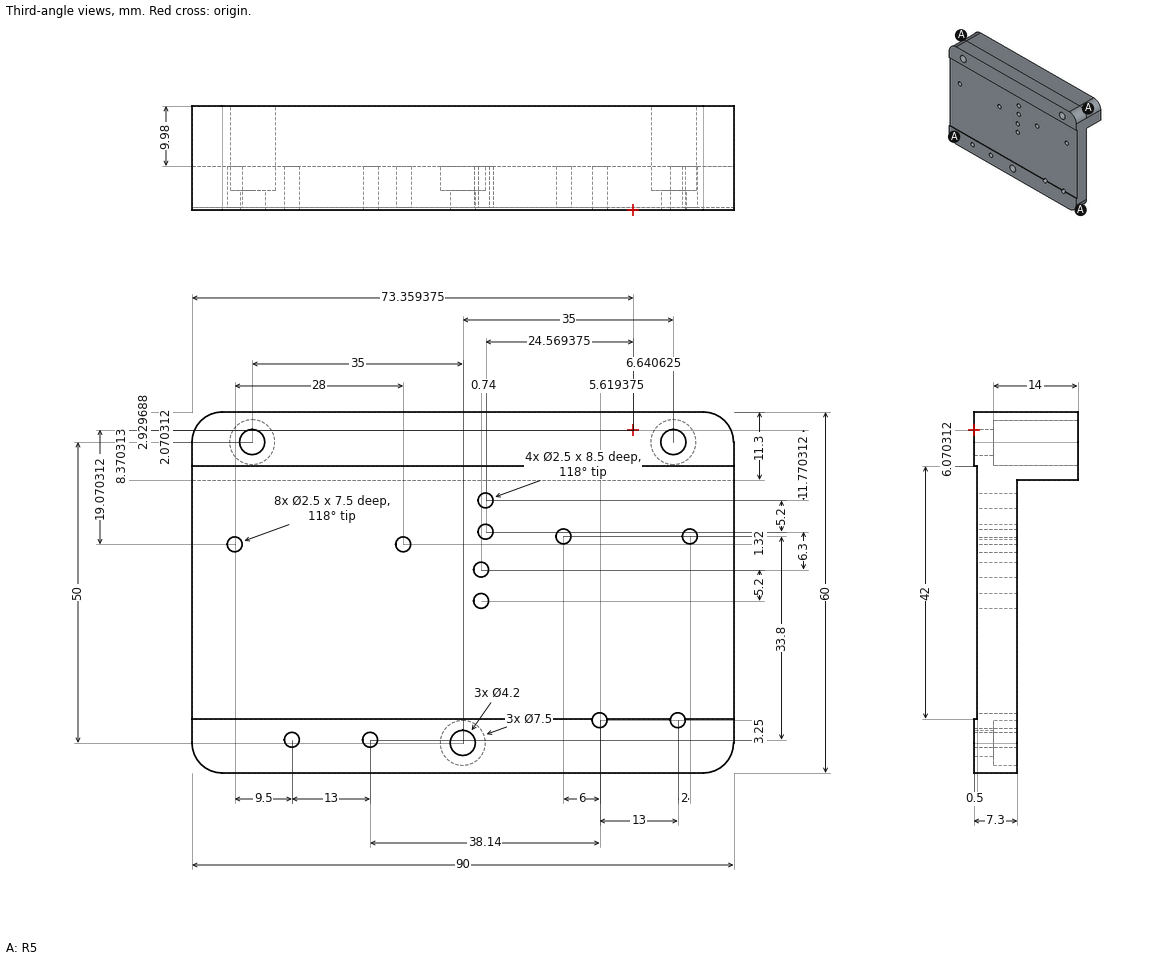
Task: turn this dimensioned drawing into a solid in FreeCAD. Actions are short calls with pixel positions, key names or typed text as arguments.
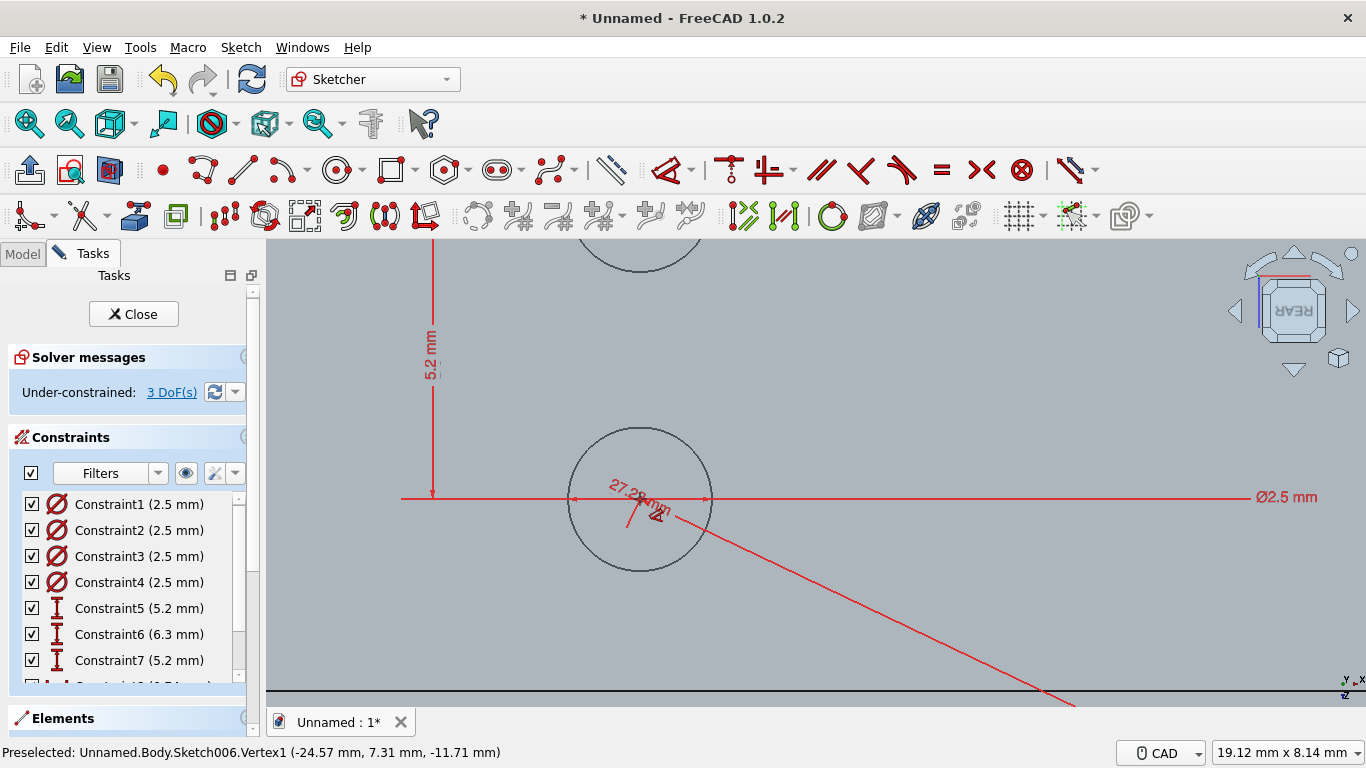
scroll(640, 504, down, 9)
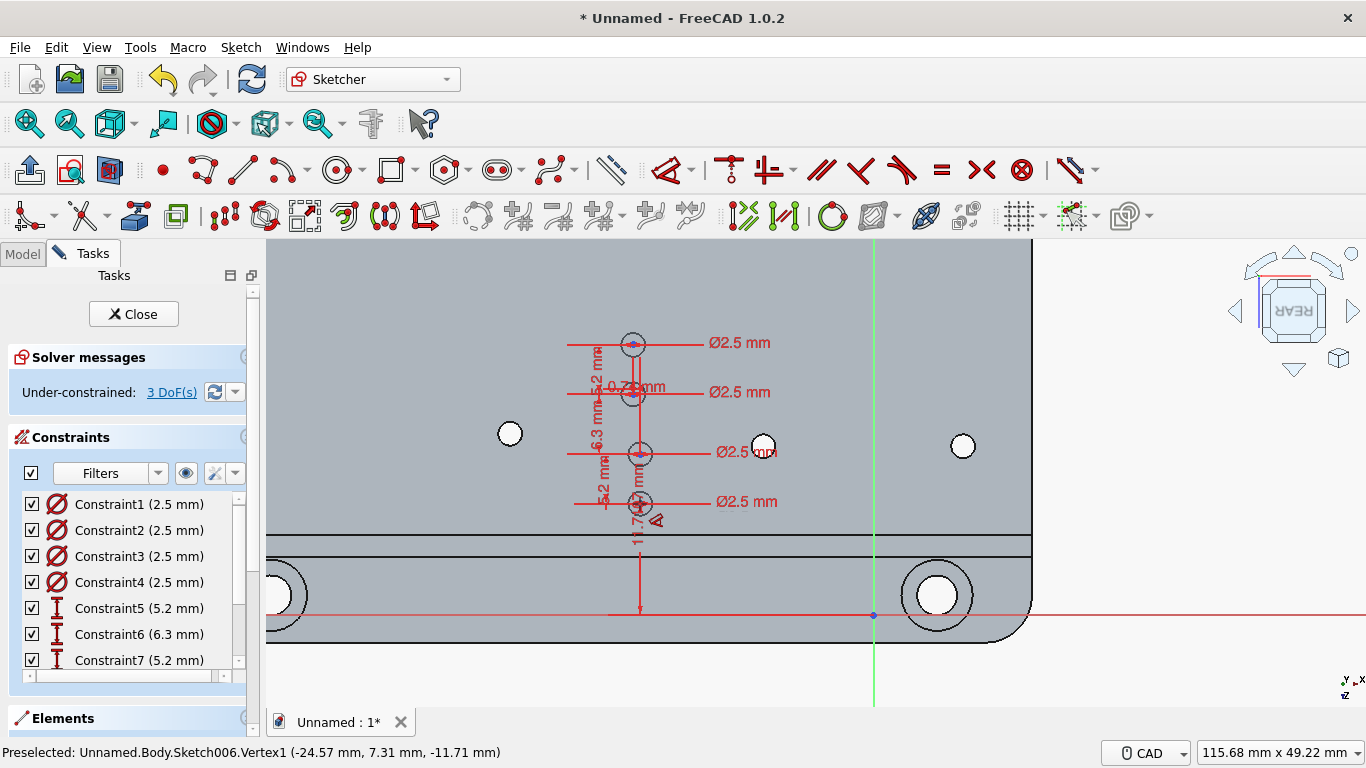
scroll(633, 394, up, 9)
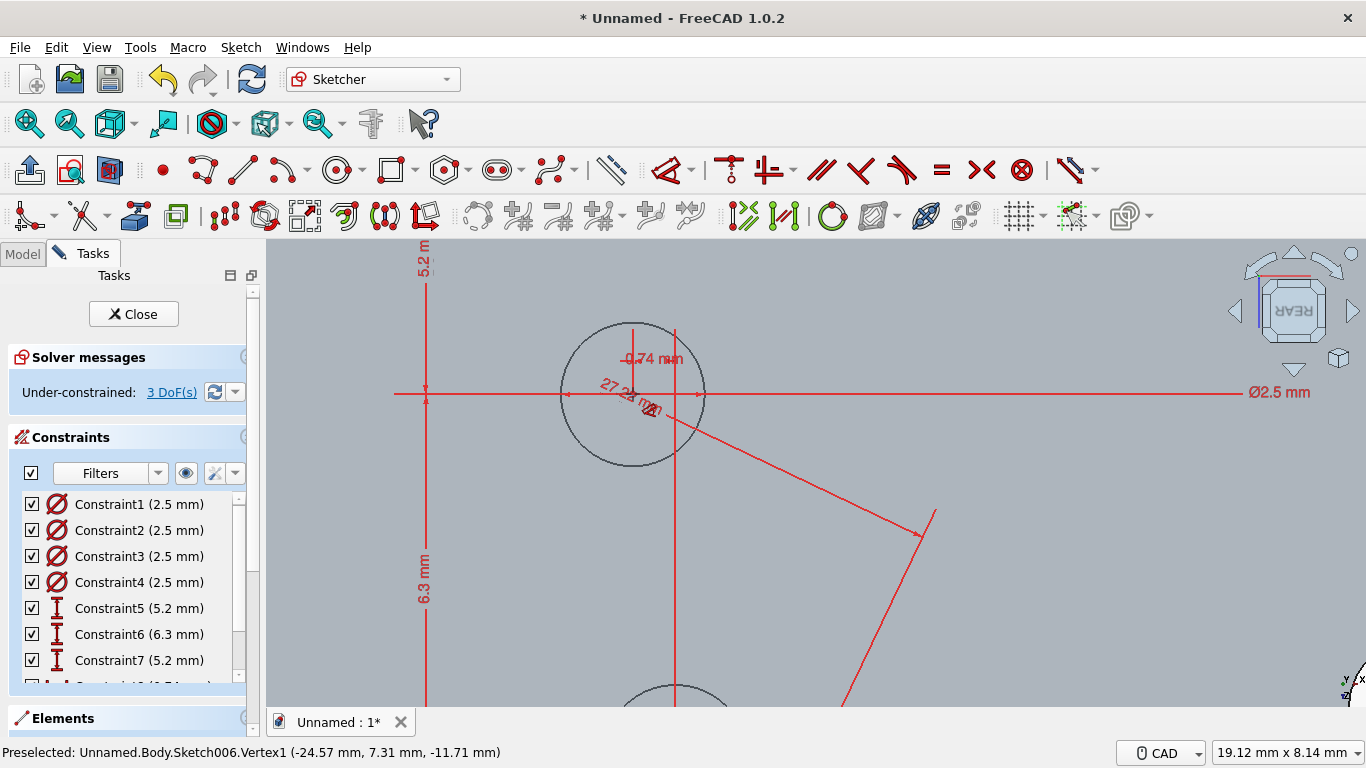
click(633, 394)
click(639, 336)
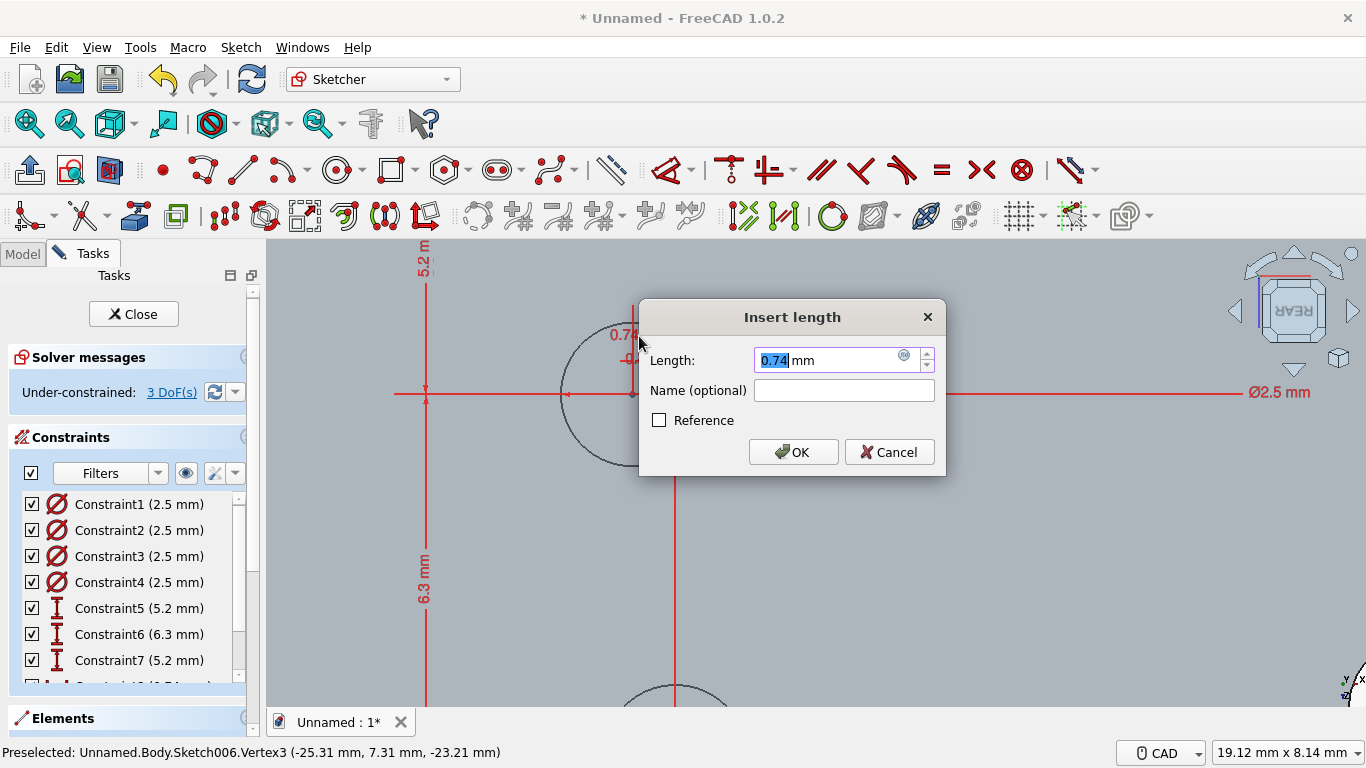
text(0.74)
key(Return)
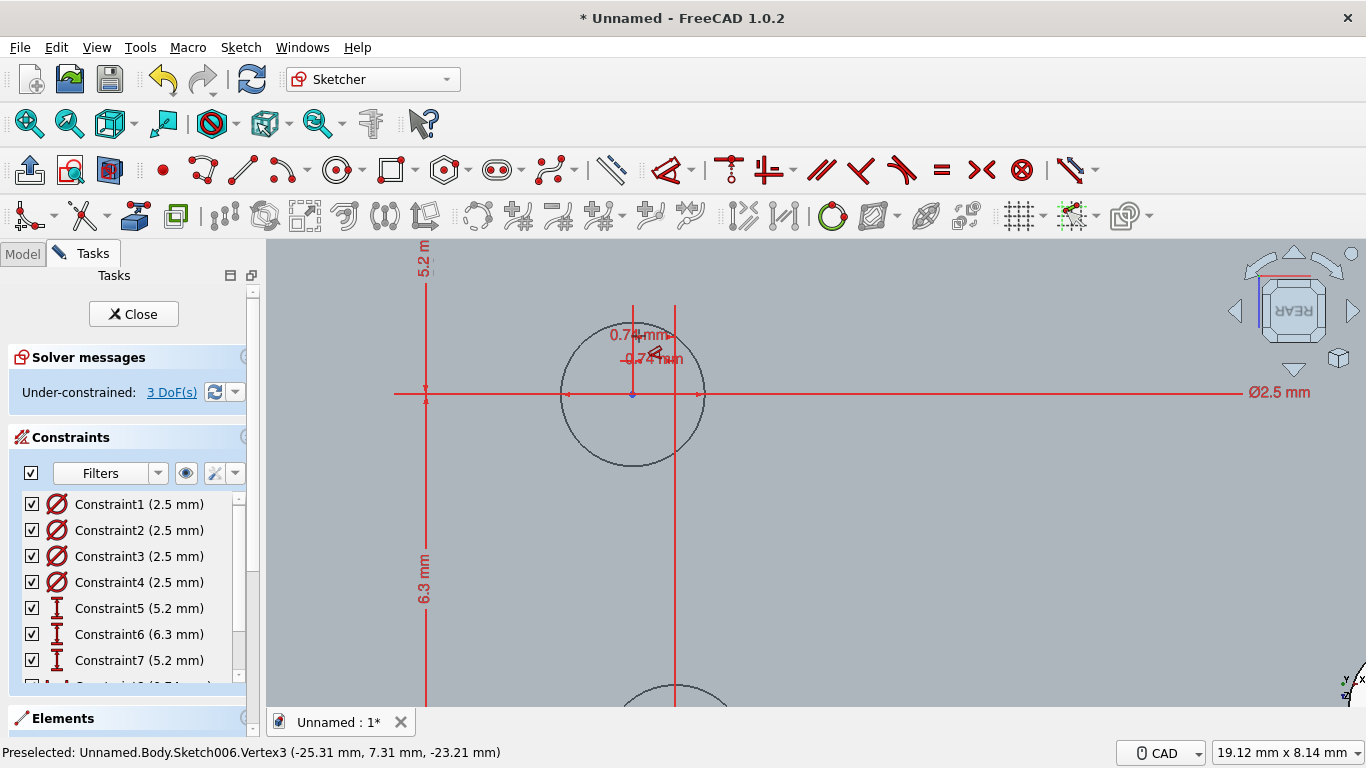
scroll(633, 393, down, 9)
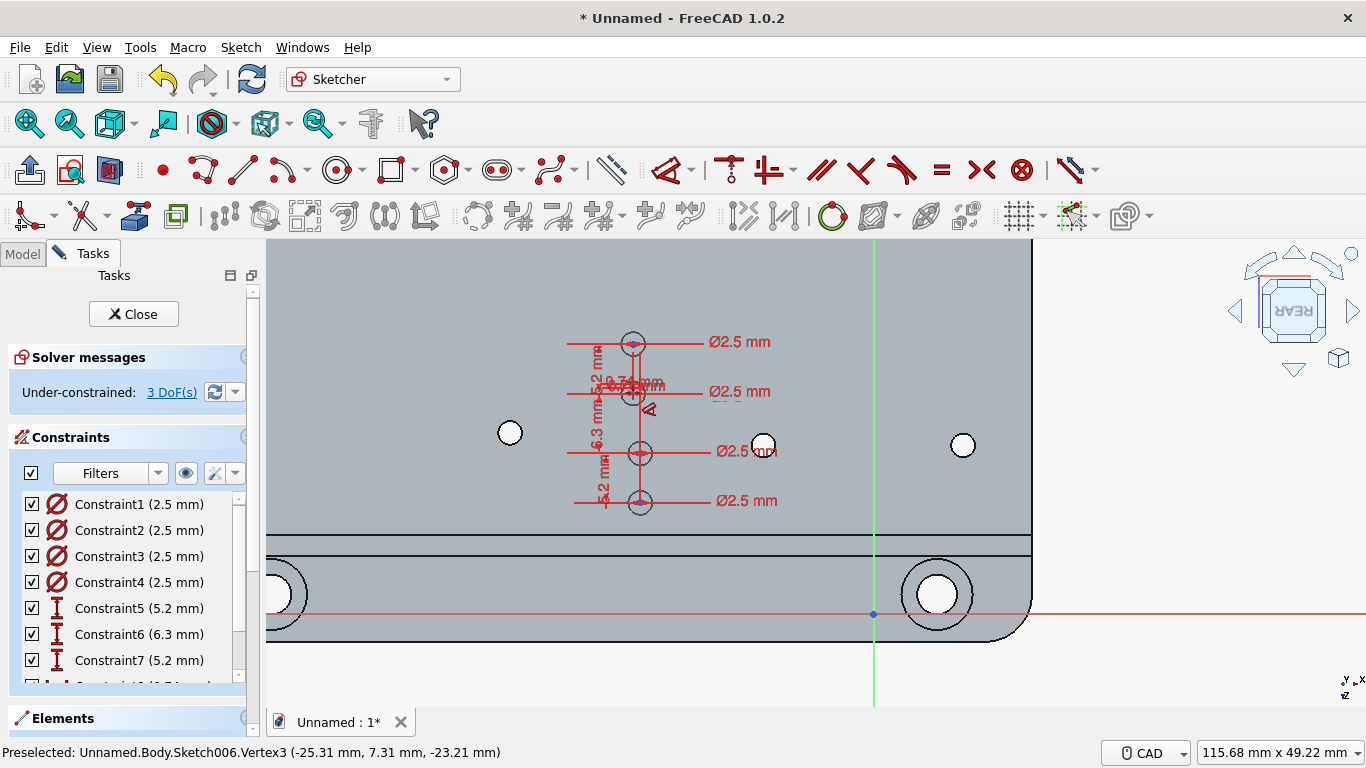
scroll(640, 453, up, 9)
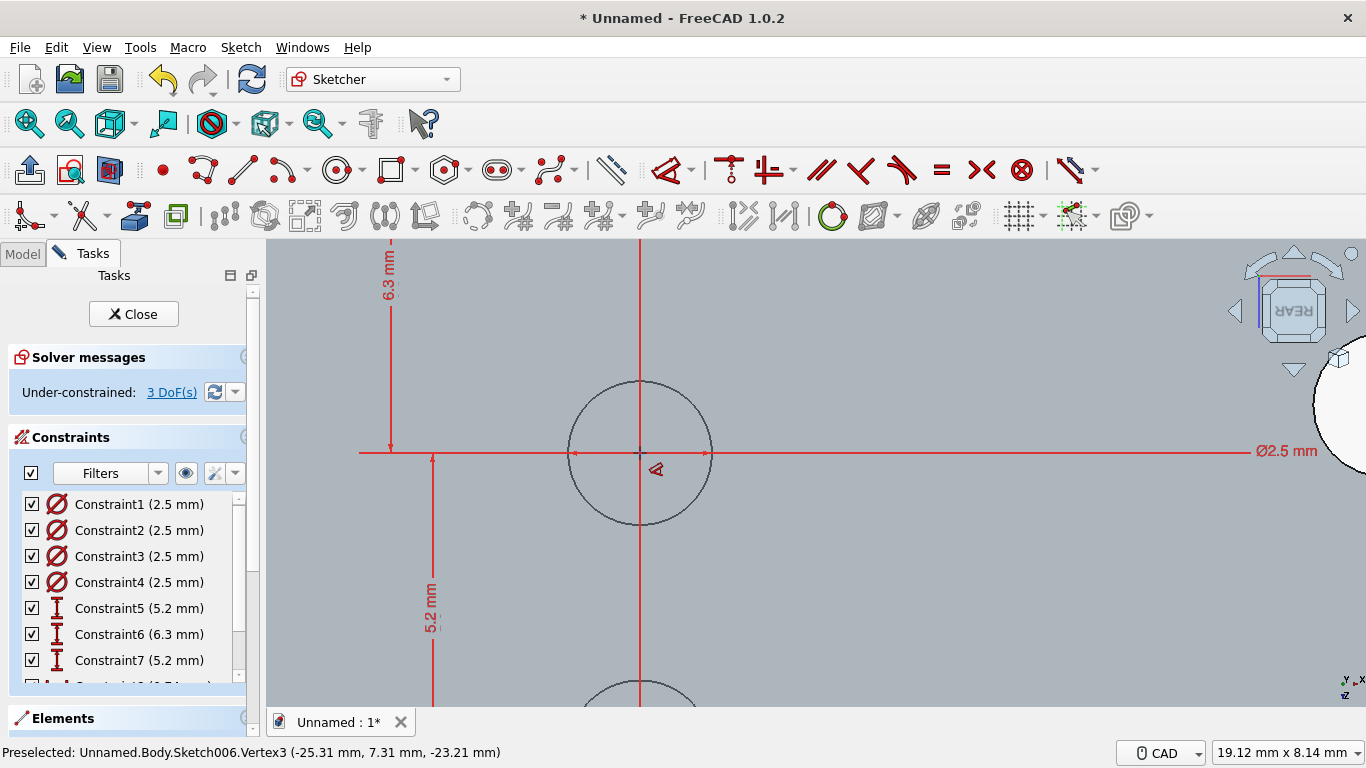
click(640, 453)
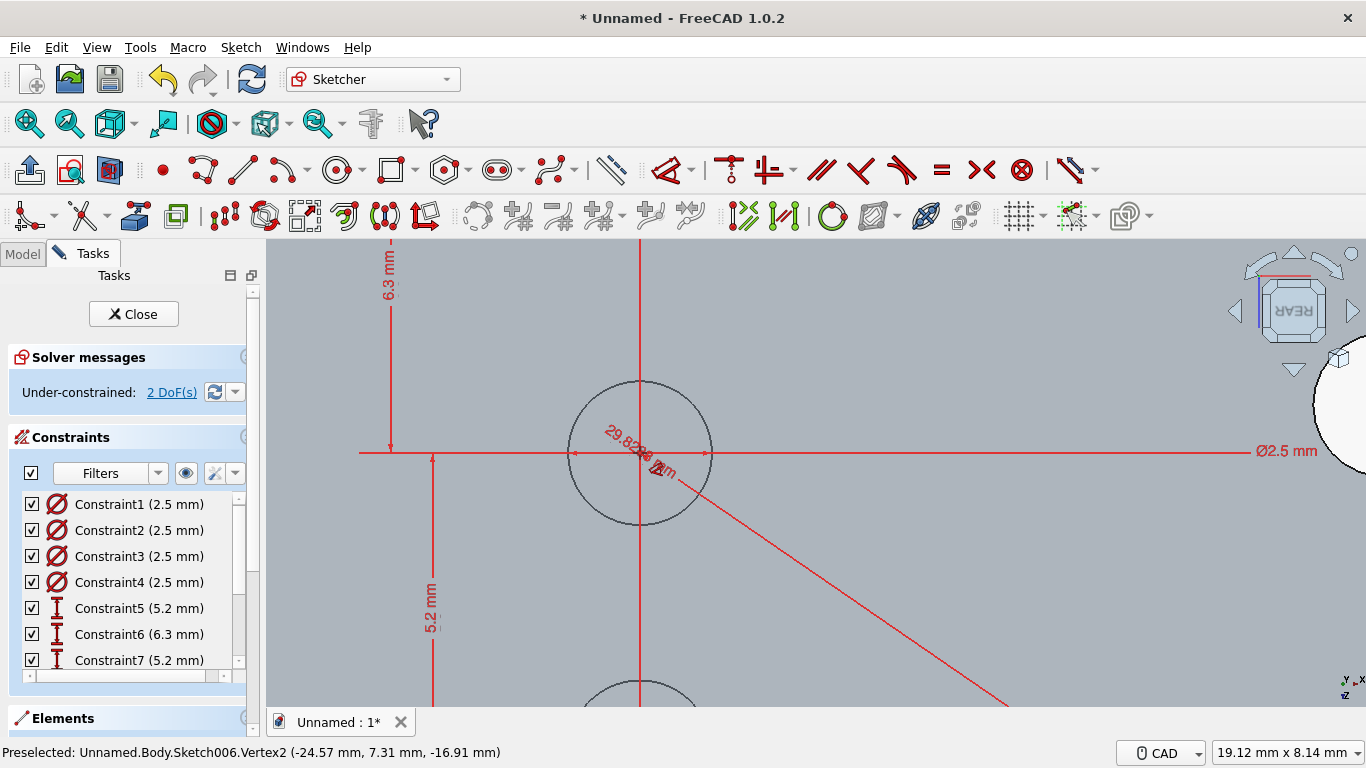
scroll(640, 454, down, 9)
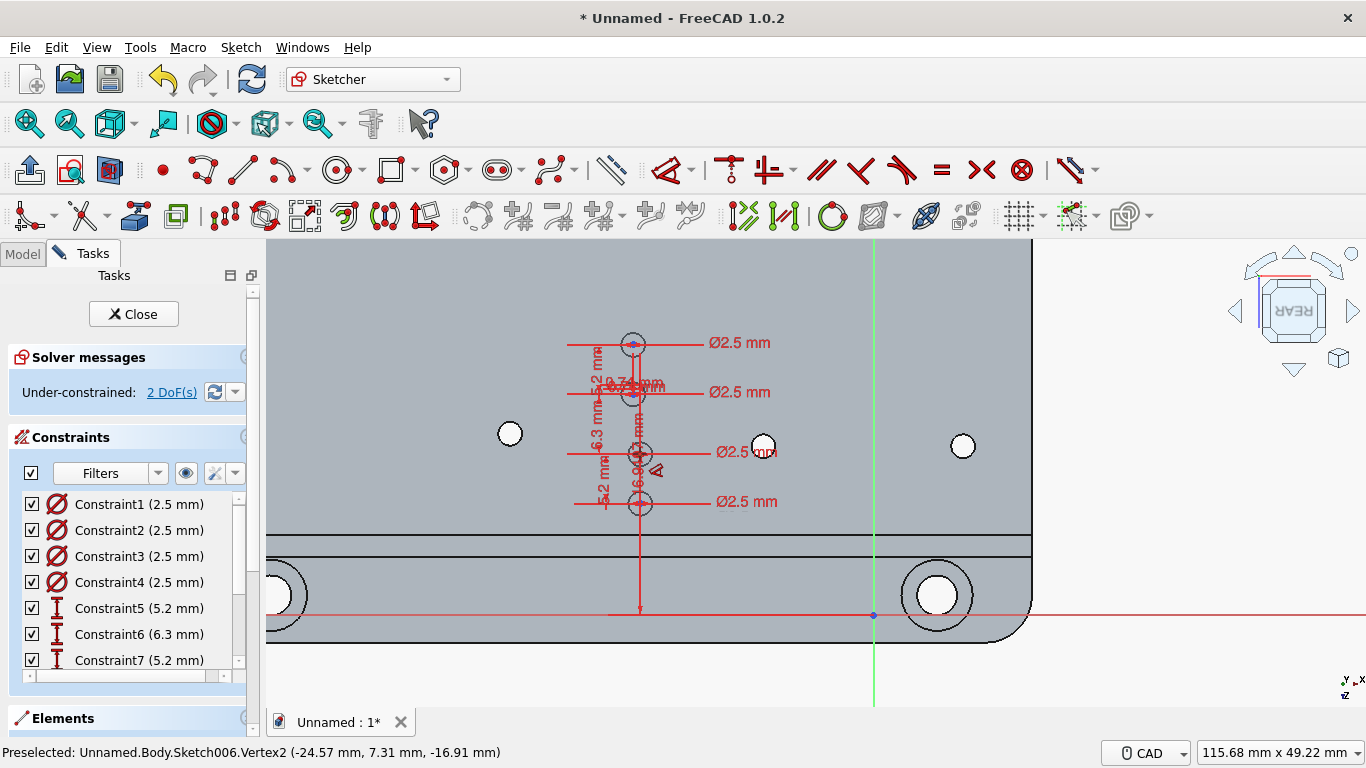
scroll(633, 345, up, 9)